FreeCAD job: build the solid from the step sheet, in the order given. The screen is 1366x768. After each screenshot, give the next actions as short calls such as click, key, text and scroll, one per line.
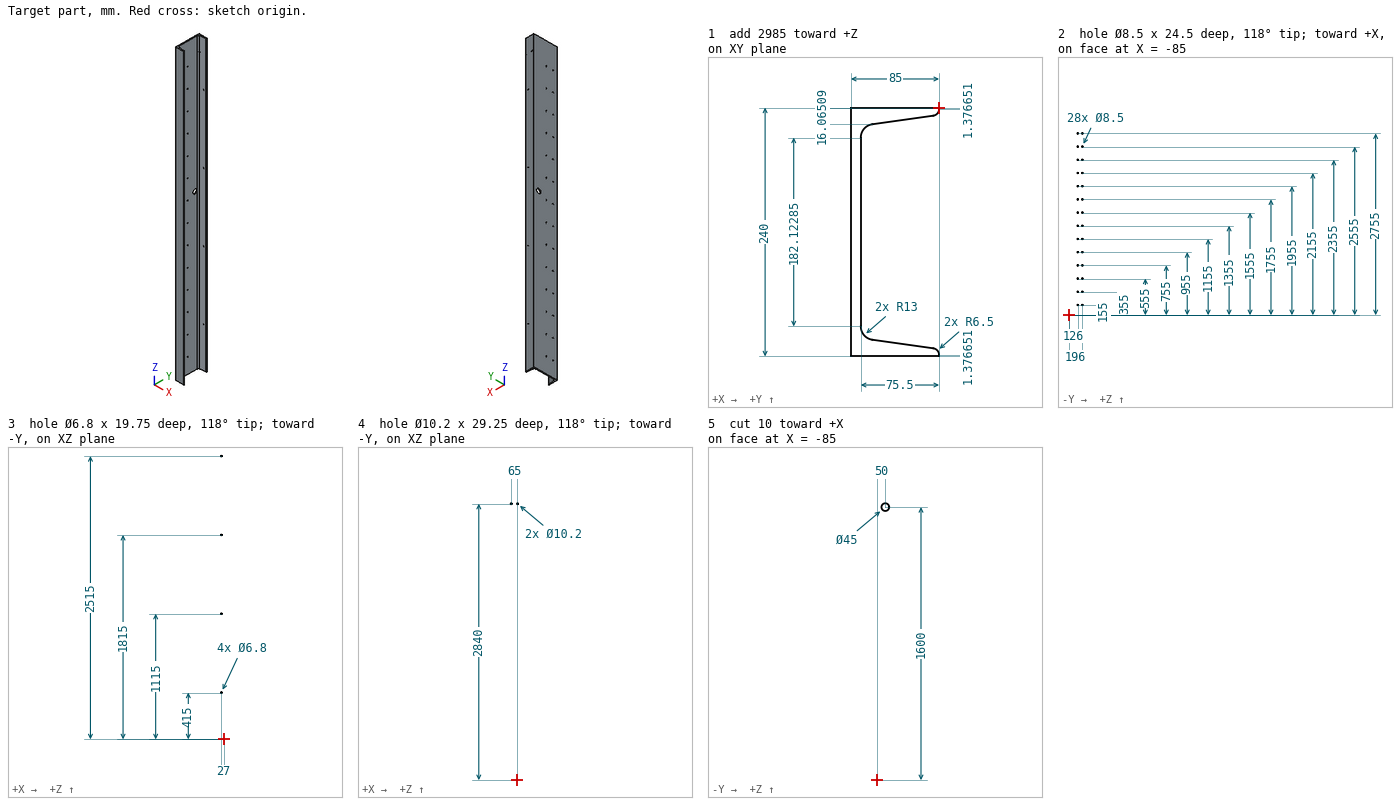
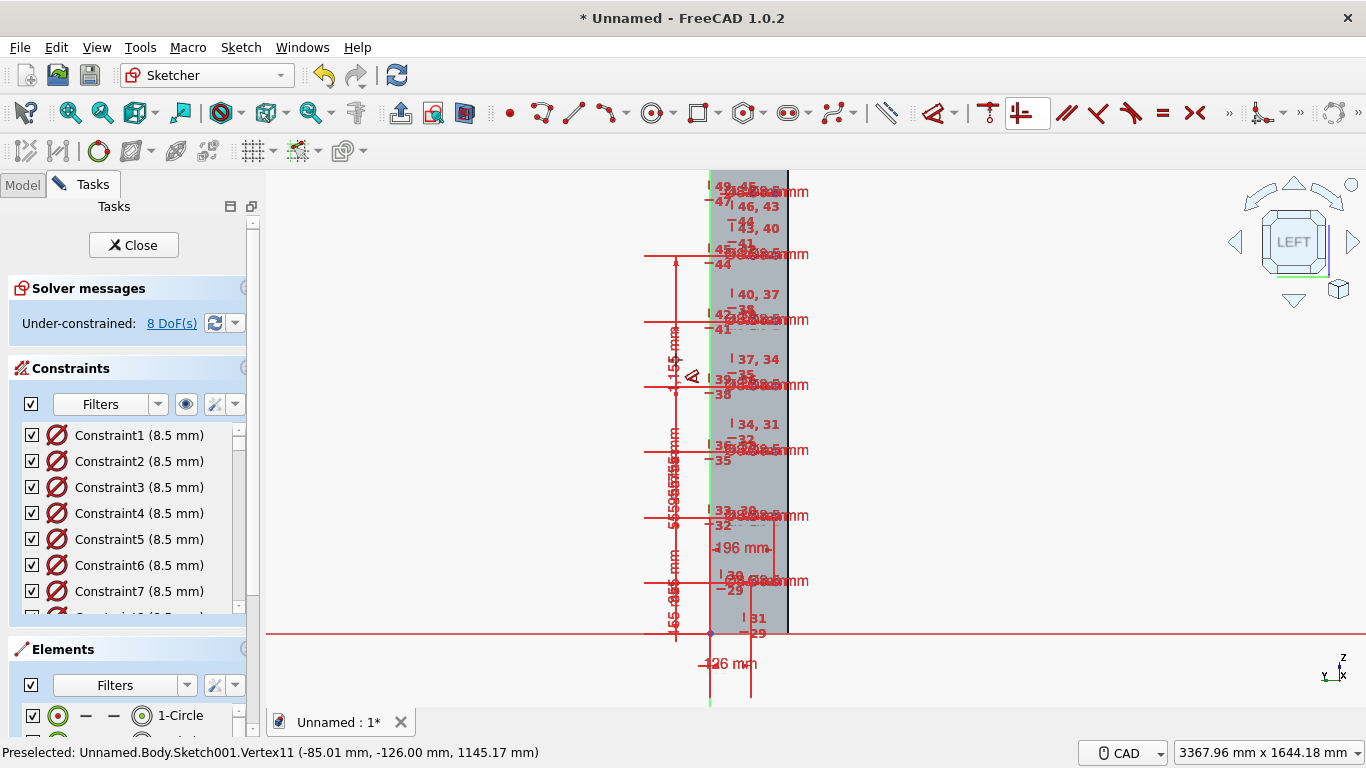
scroll(750, 587, down, 5)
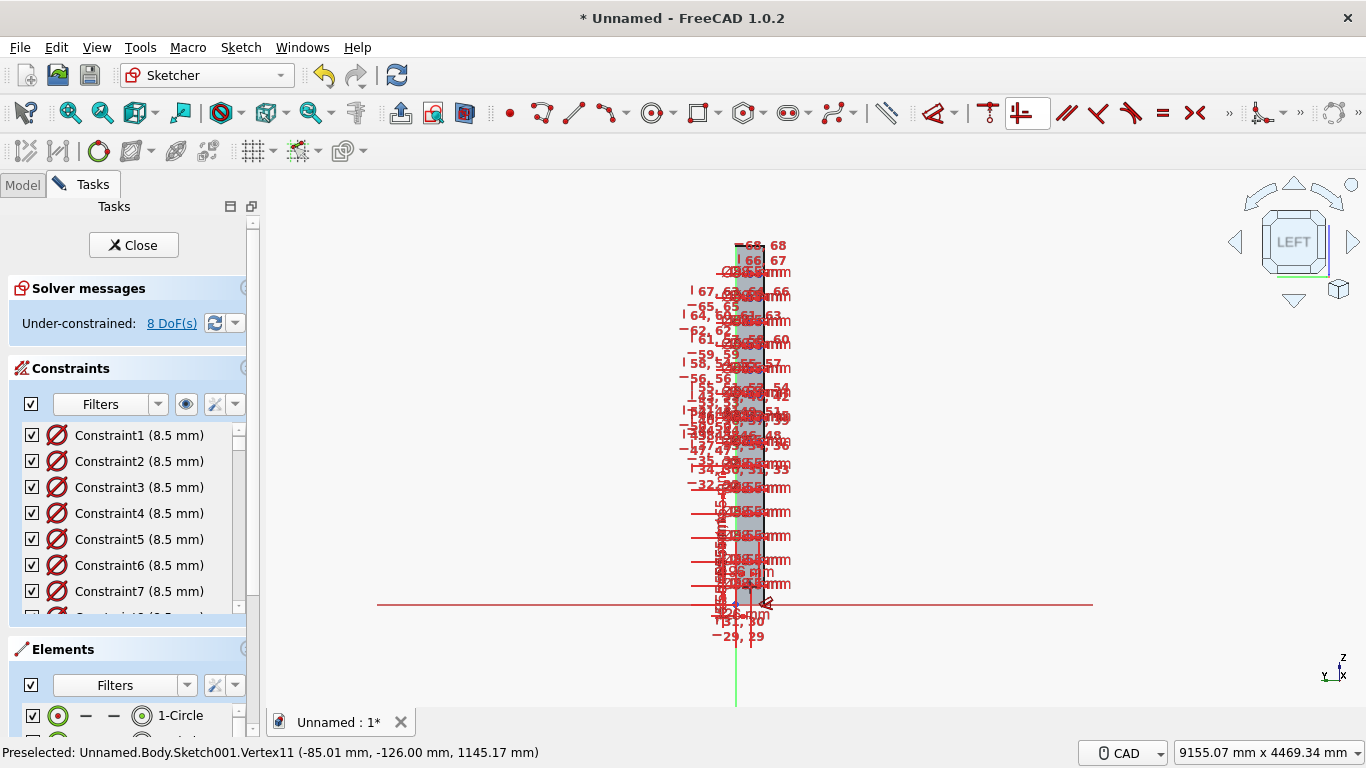
scroll(751, 443, up, 2)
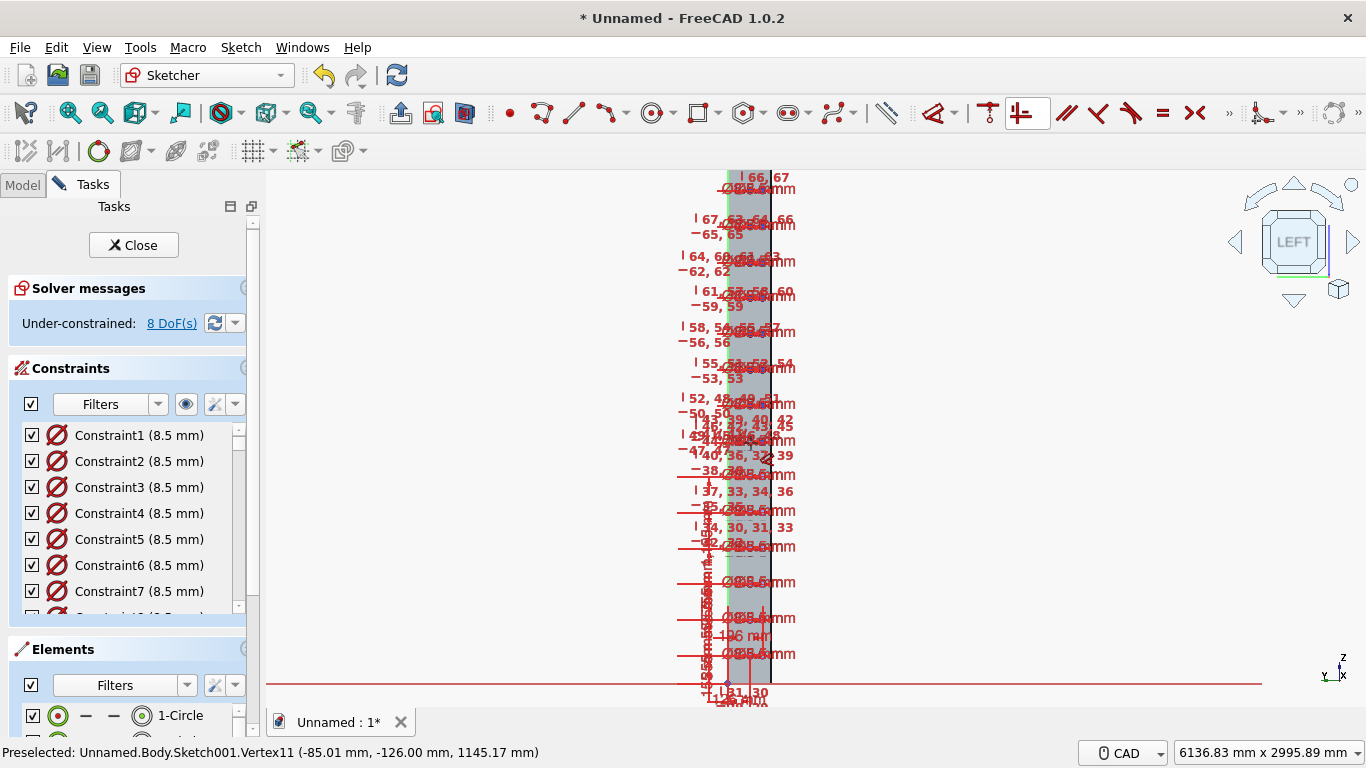
click(750, 443)
click(694, 561)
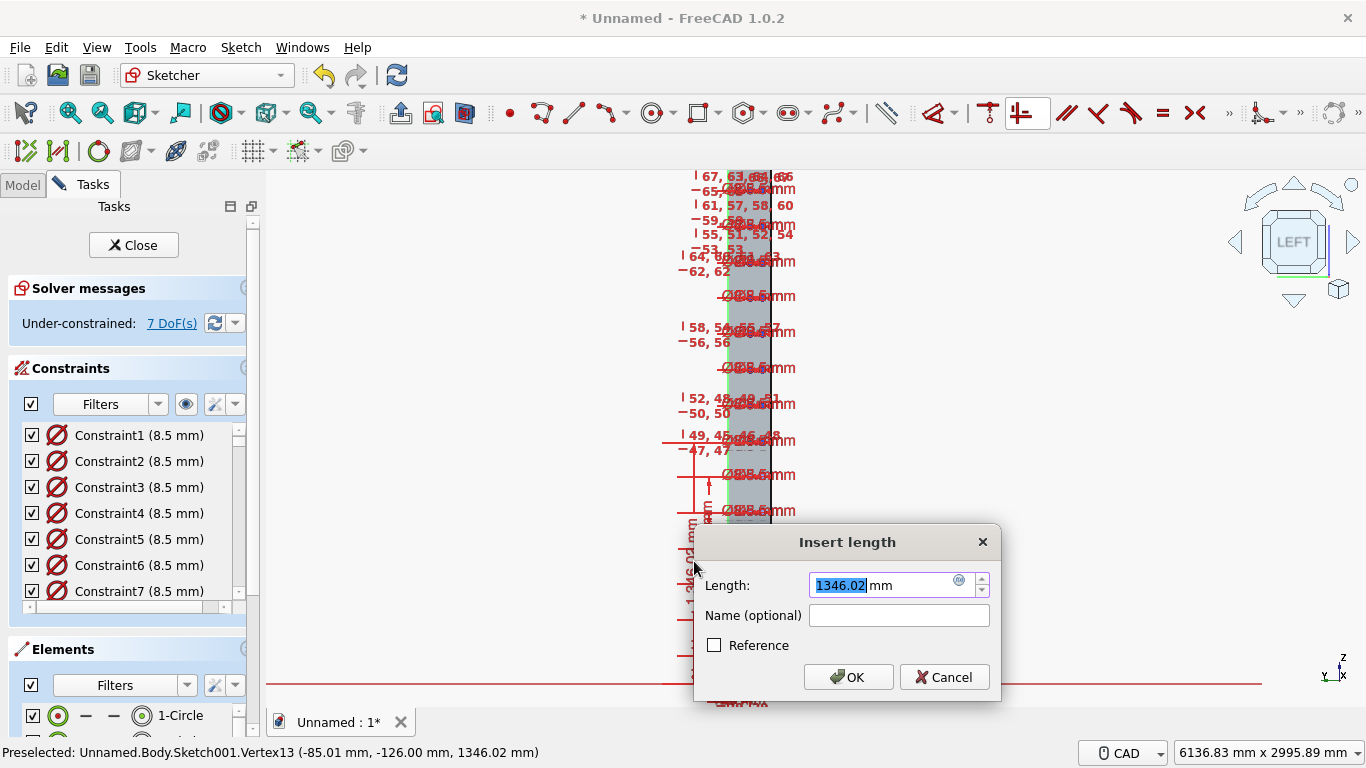
text(1355)
key(Return)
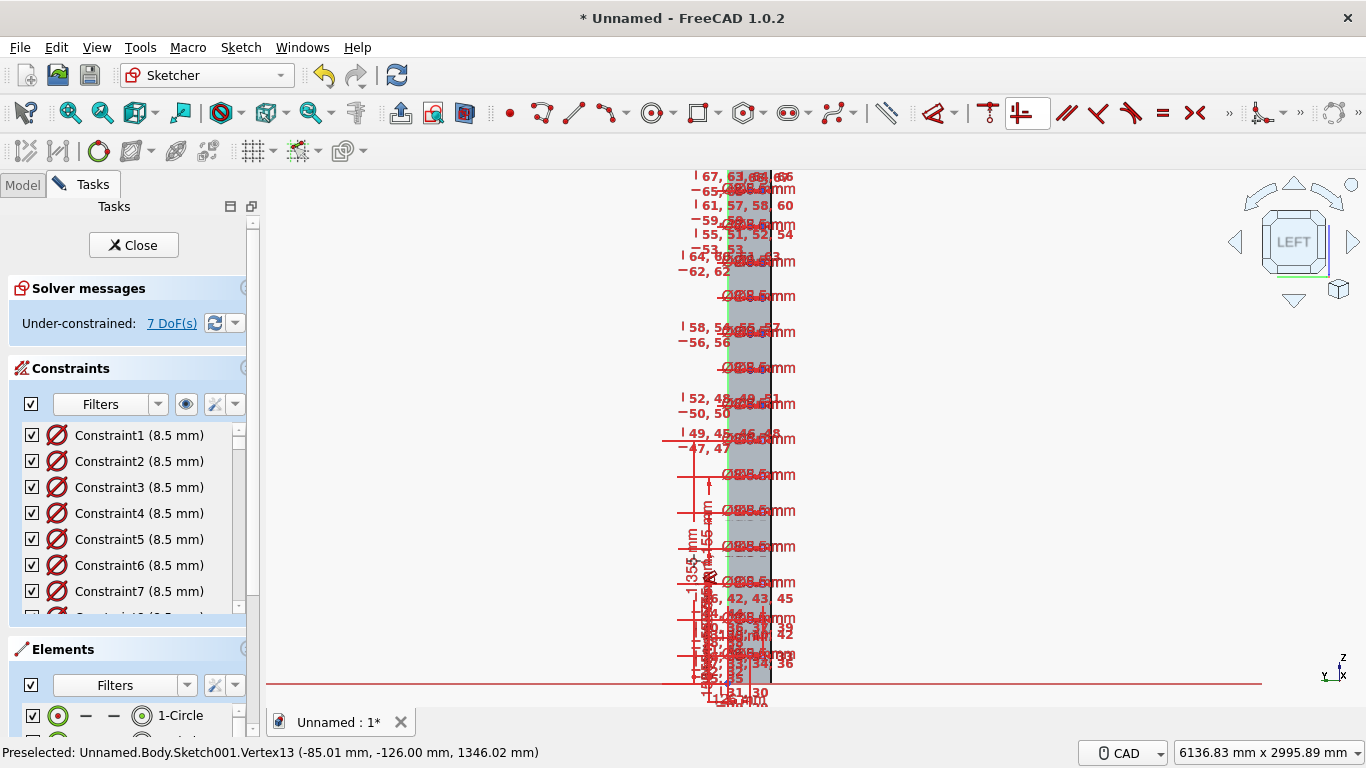
click(763, 406)
click(694, 480)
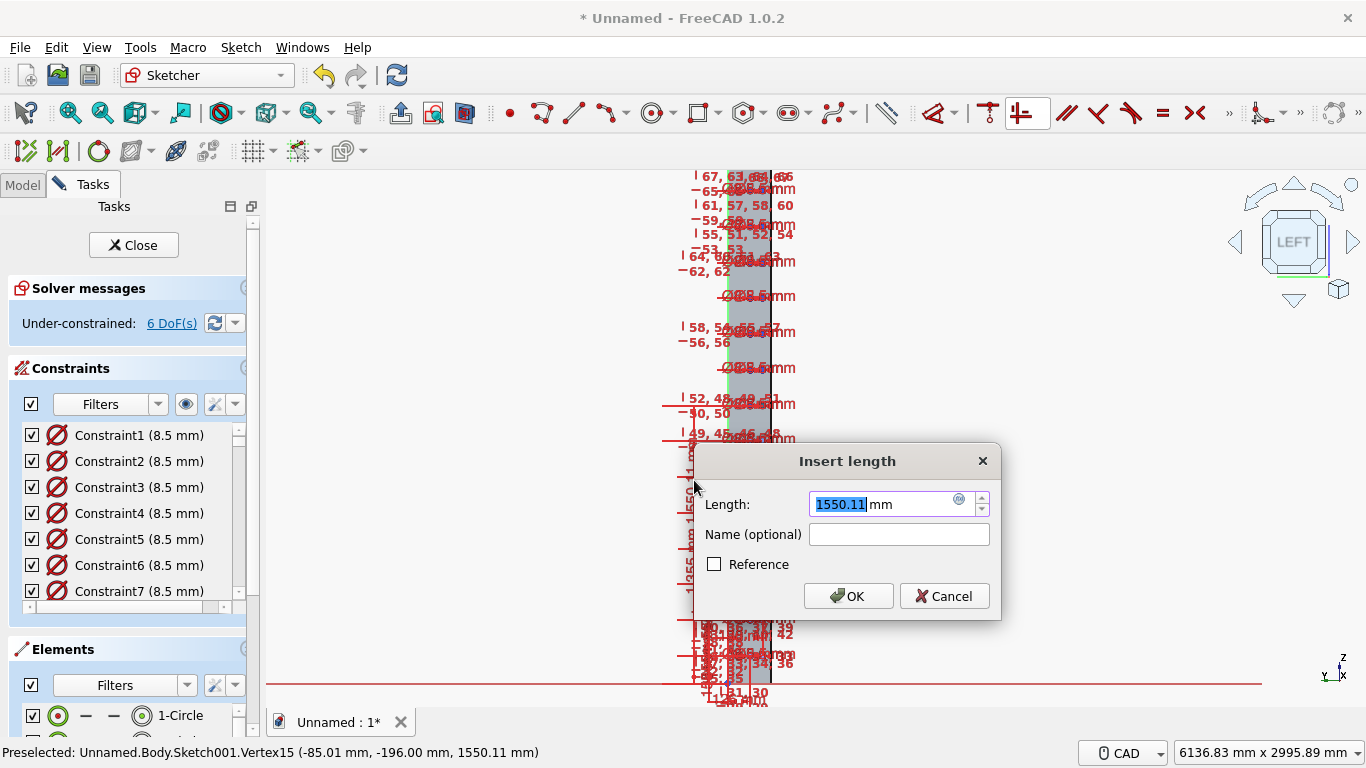
text(1555)
key(Return)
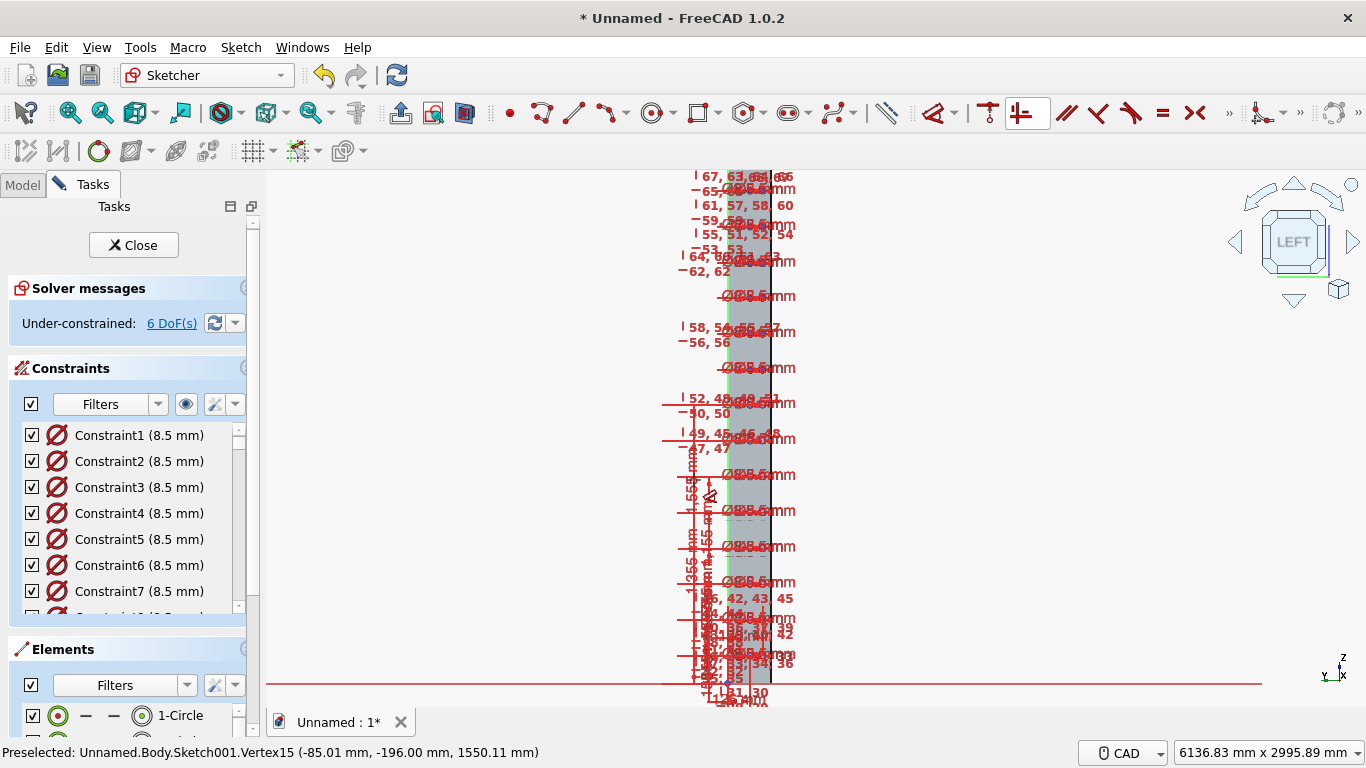
click(763, 370)
click(694, 453)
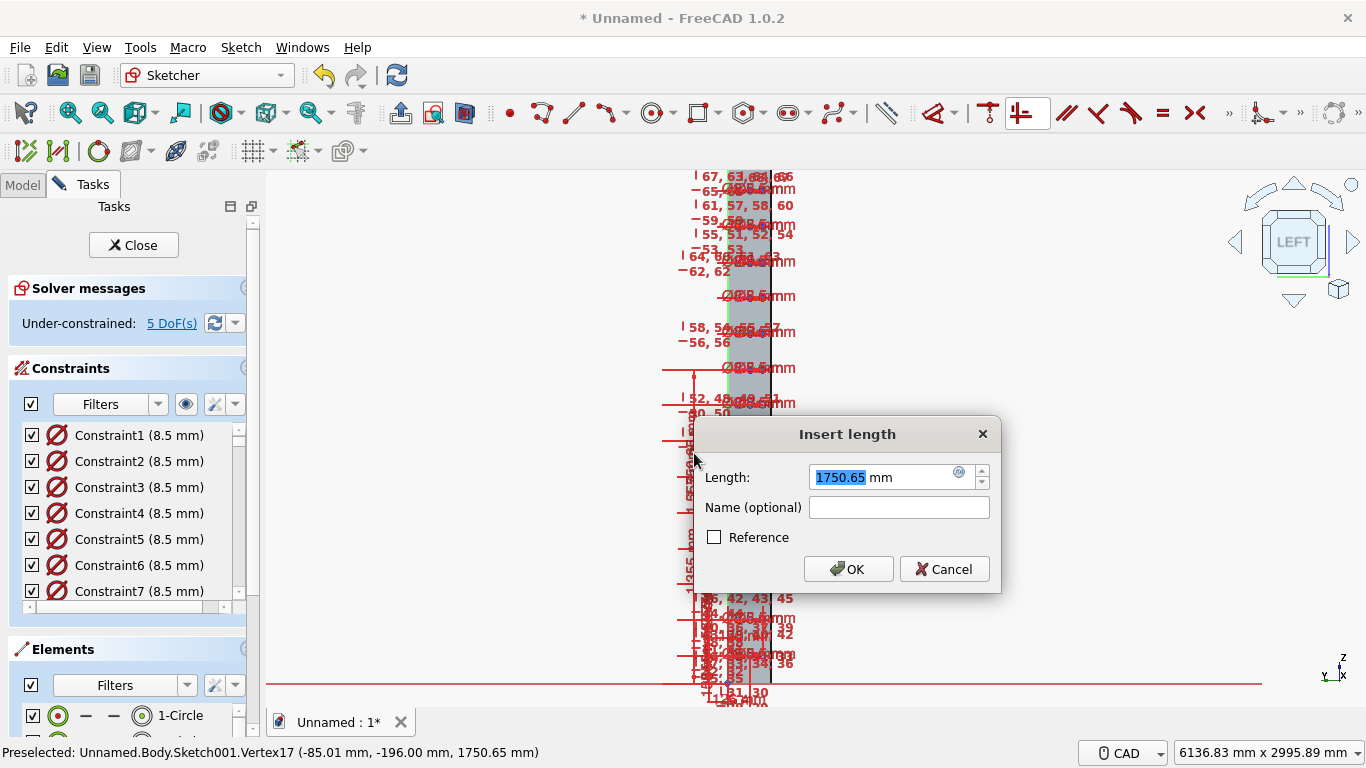
text(1755)
key(Return)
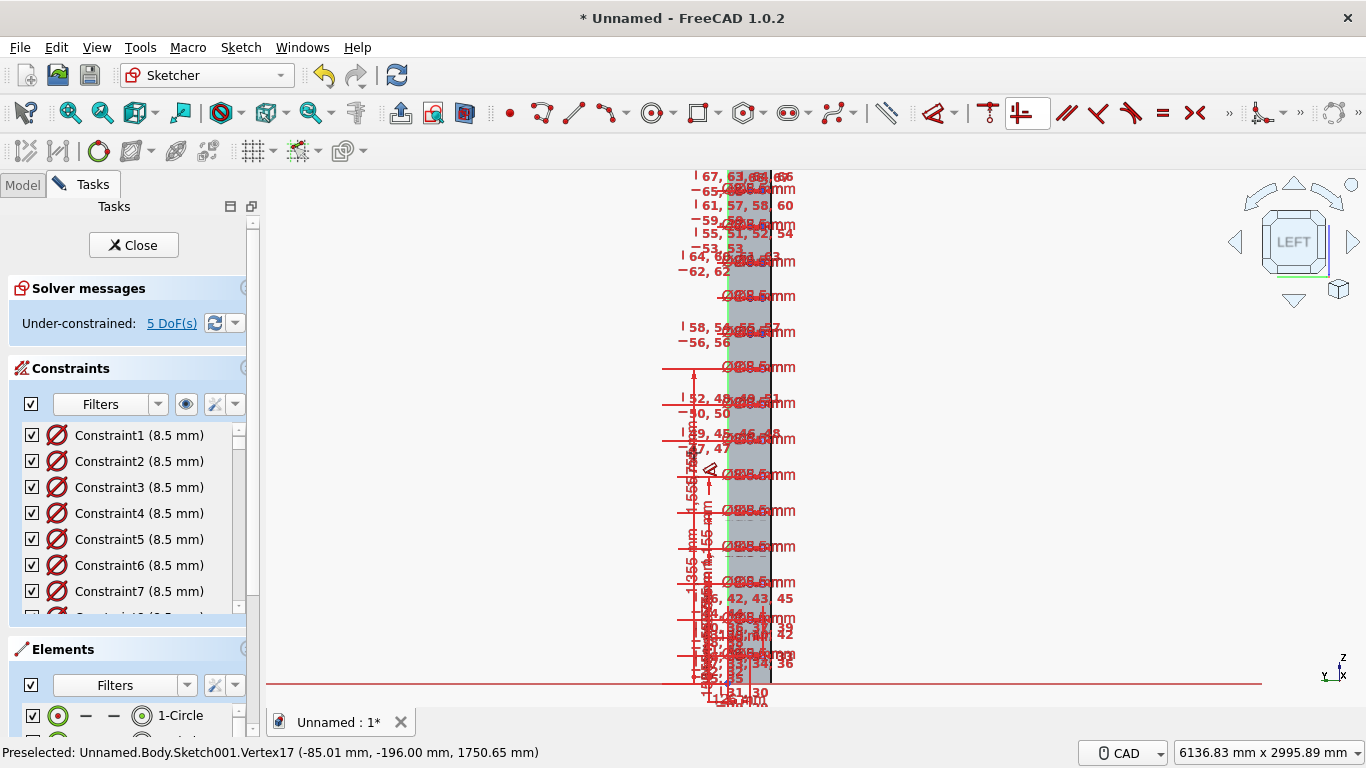
click(750, 334)
click(694, 507)